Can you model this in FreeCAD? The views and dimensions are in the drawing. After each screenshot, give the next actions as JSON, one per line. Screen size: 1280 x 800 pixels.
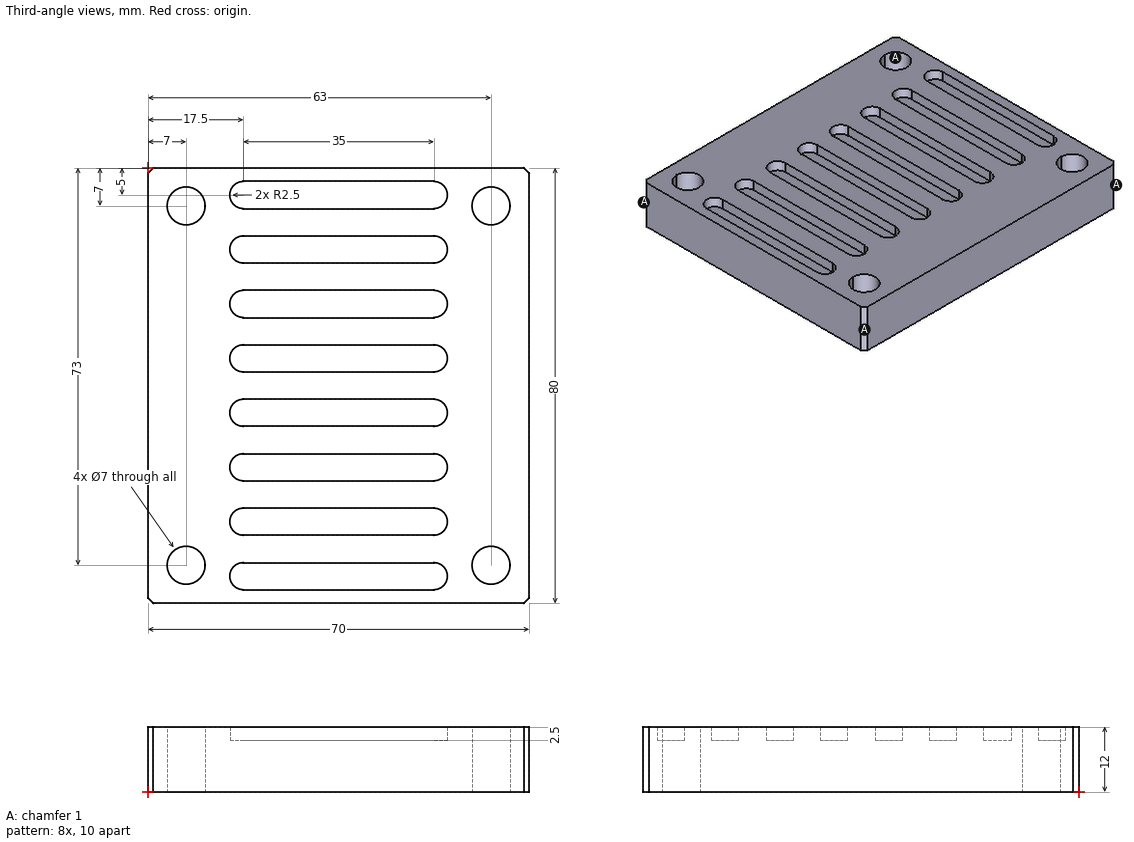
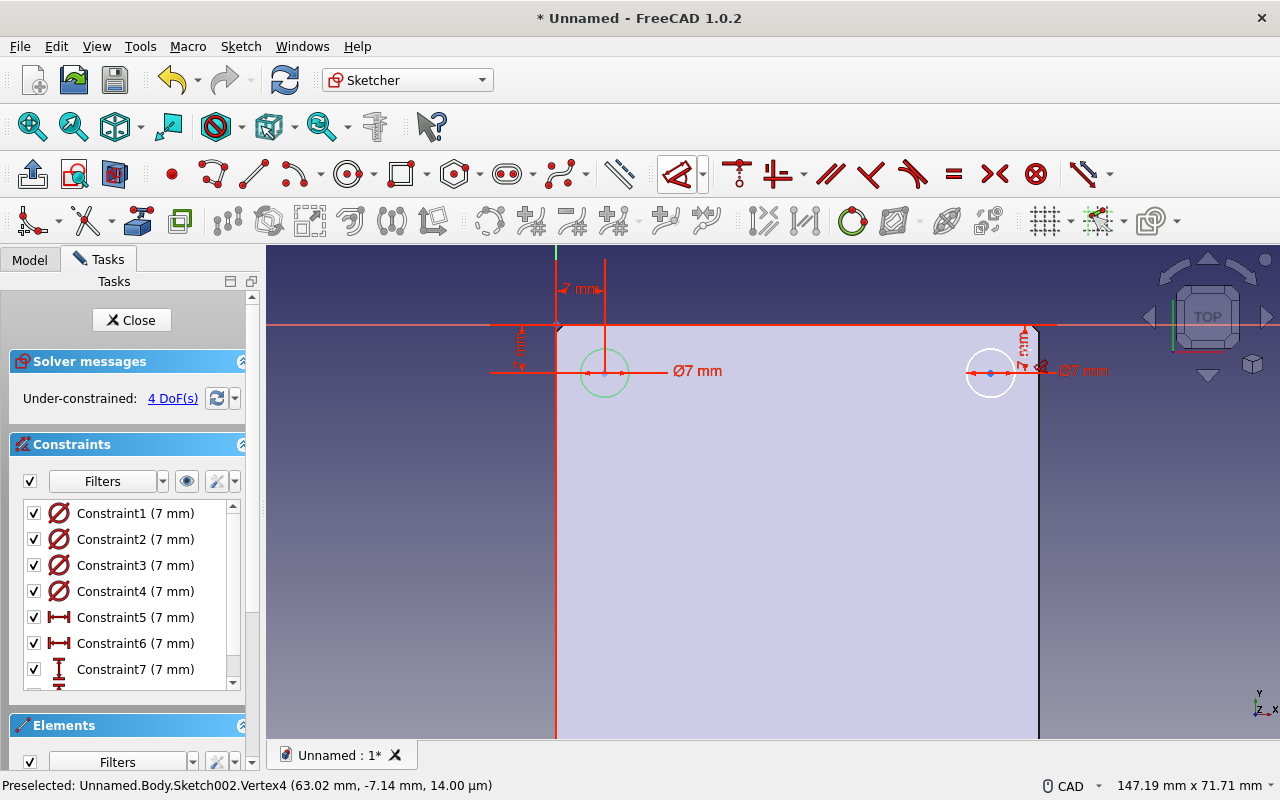
{"action": "scroll", "coordinate": [606, 375], "scroll_direction": "down", "scroll_amount": 3}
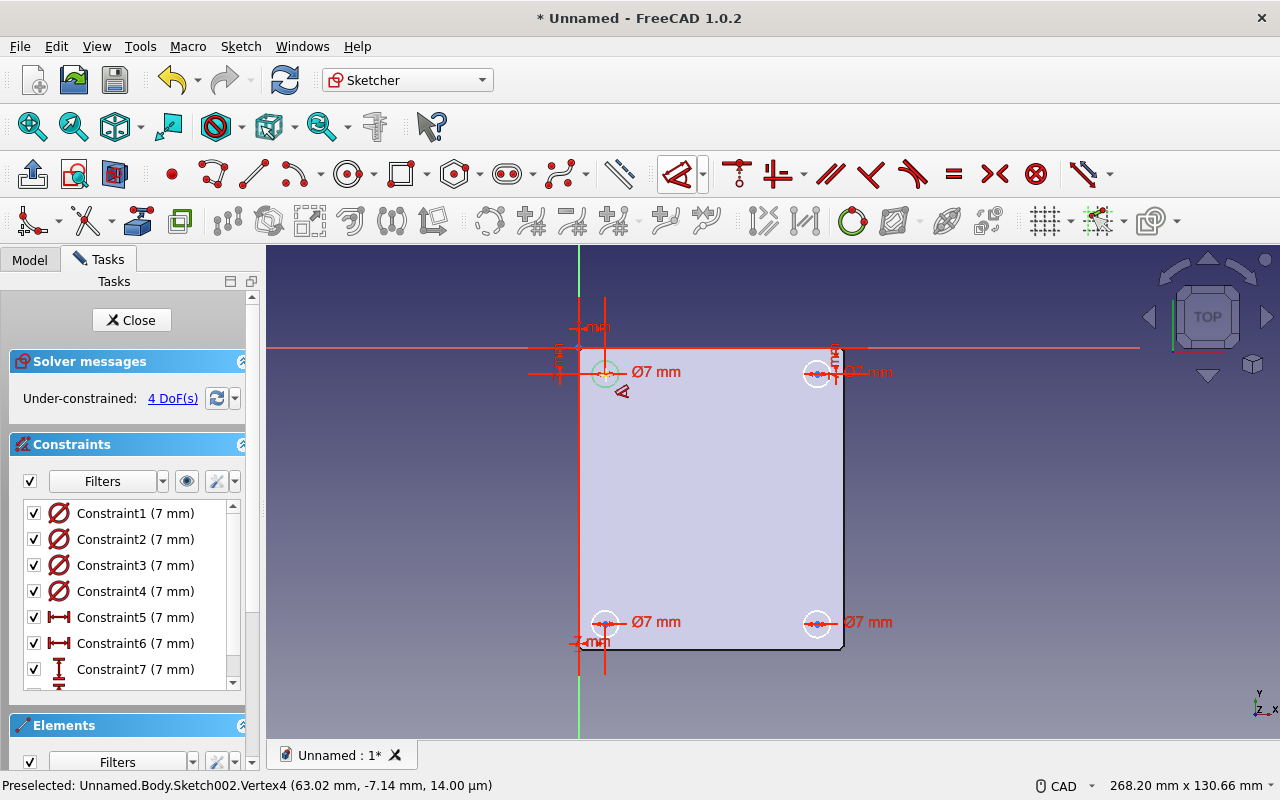
{"action": "left_click", "coordinate": [605, 624]}
{"action": "left_click", "coordinate": [545, 486]}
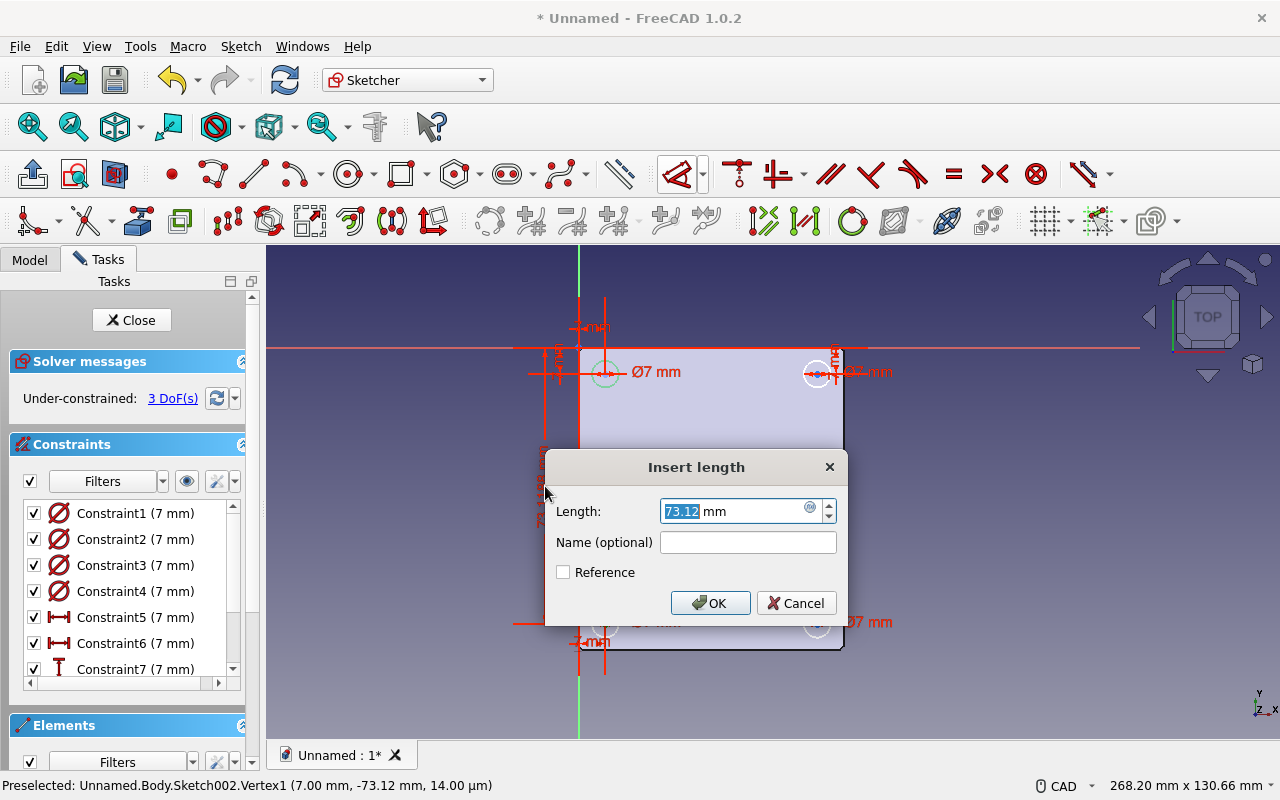
{"action": "type", "text": "73"}
{"action": "key", "text": "Return"}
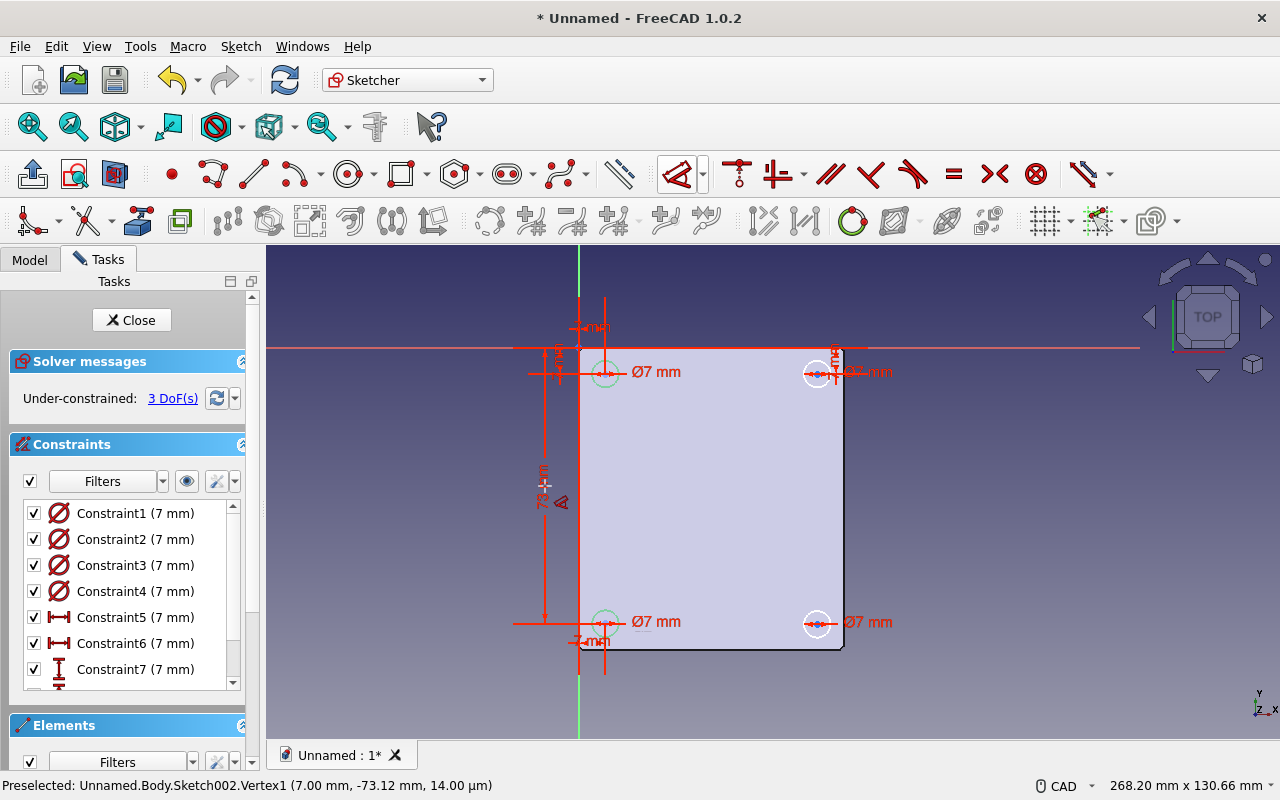
{"action": "left_click", "coordinate": [817, 624]}
{"action": "left_click", "coordinate": [698, 314]}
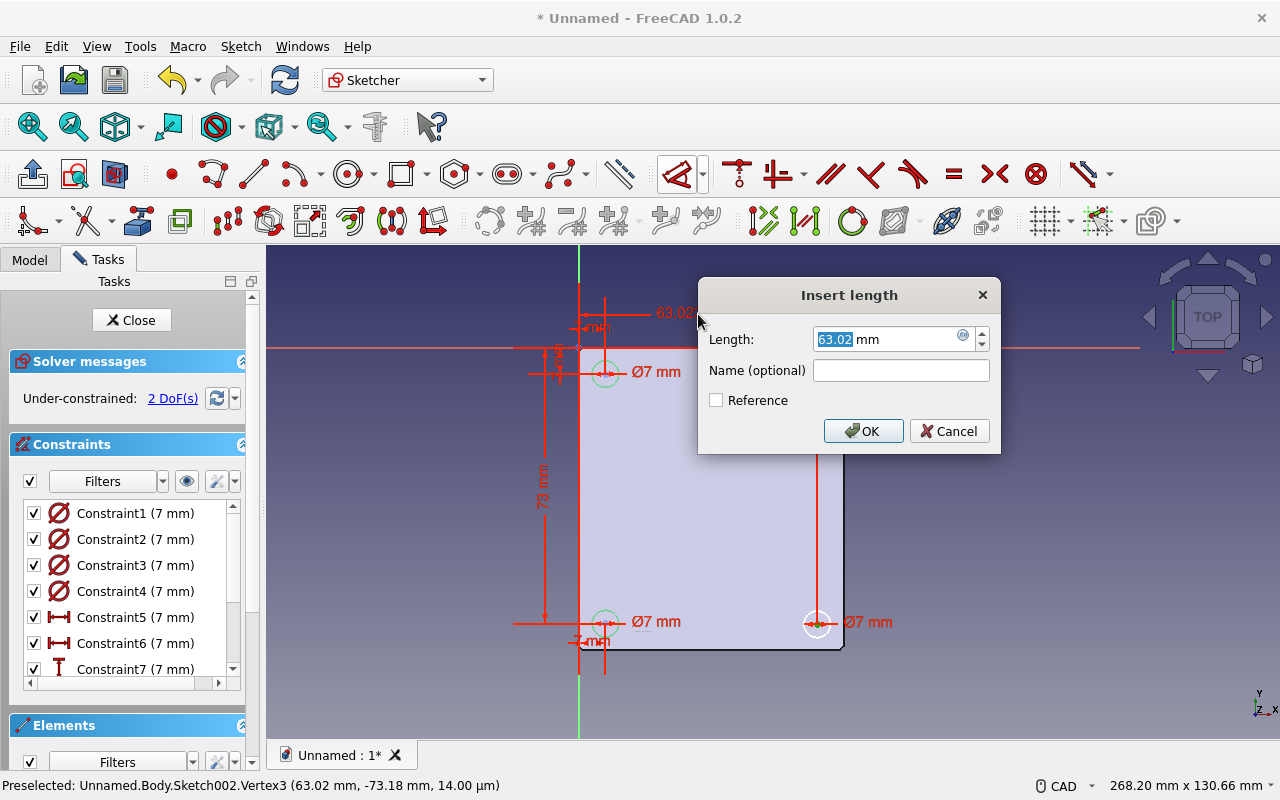
{"action": "type", "text": "63"}
{"action": "key", "text": "Return"}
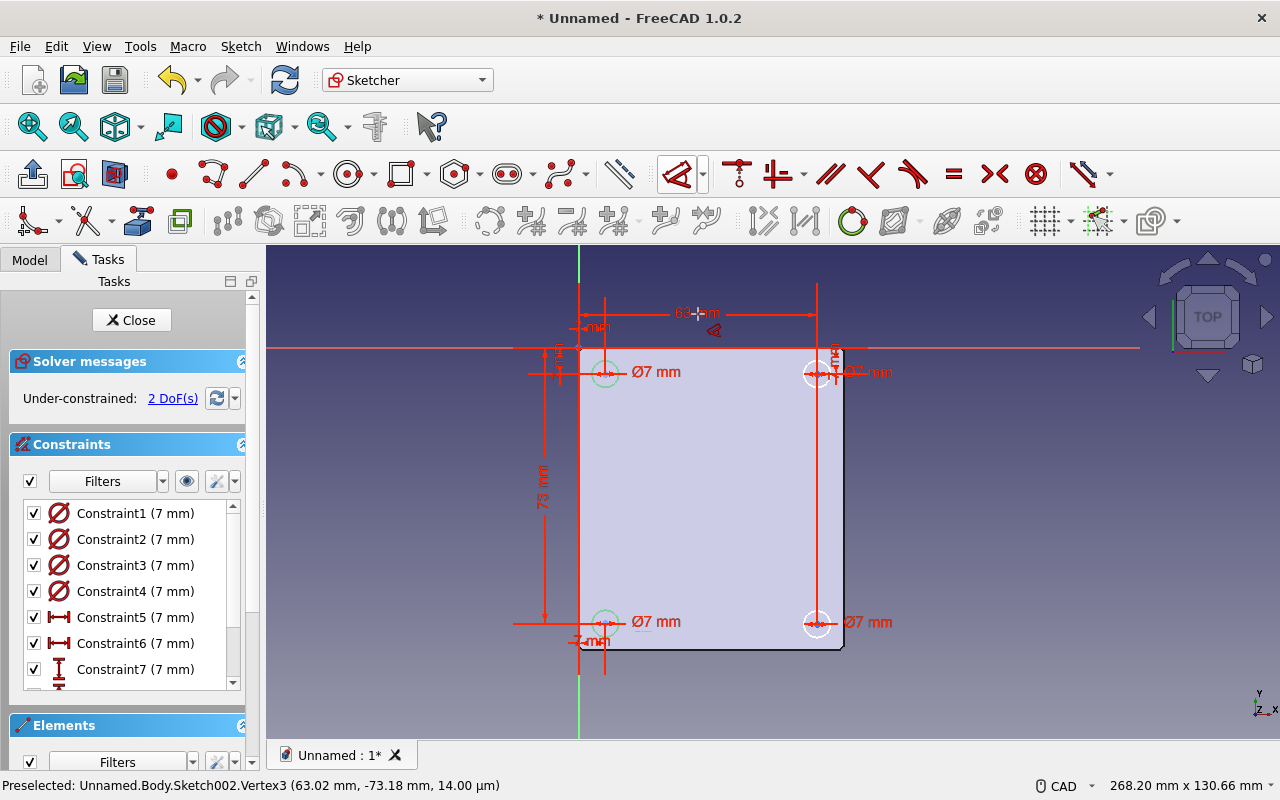
{"action": "left_click", "coordinate": [817, 624]}
{"action": "left_click", "coordinate": [545, 422]}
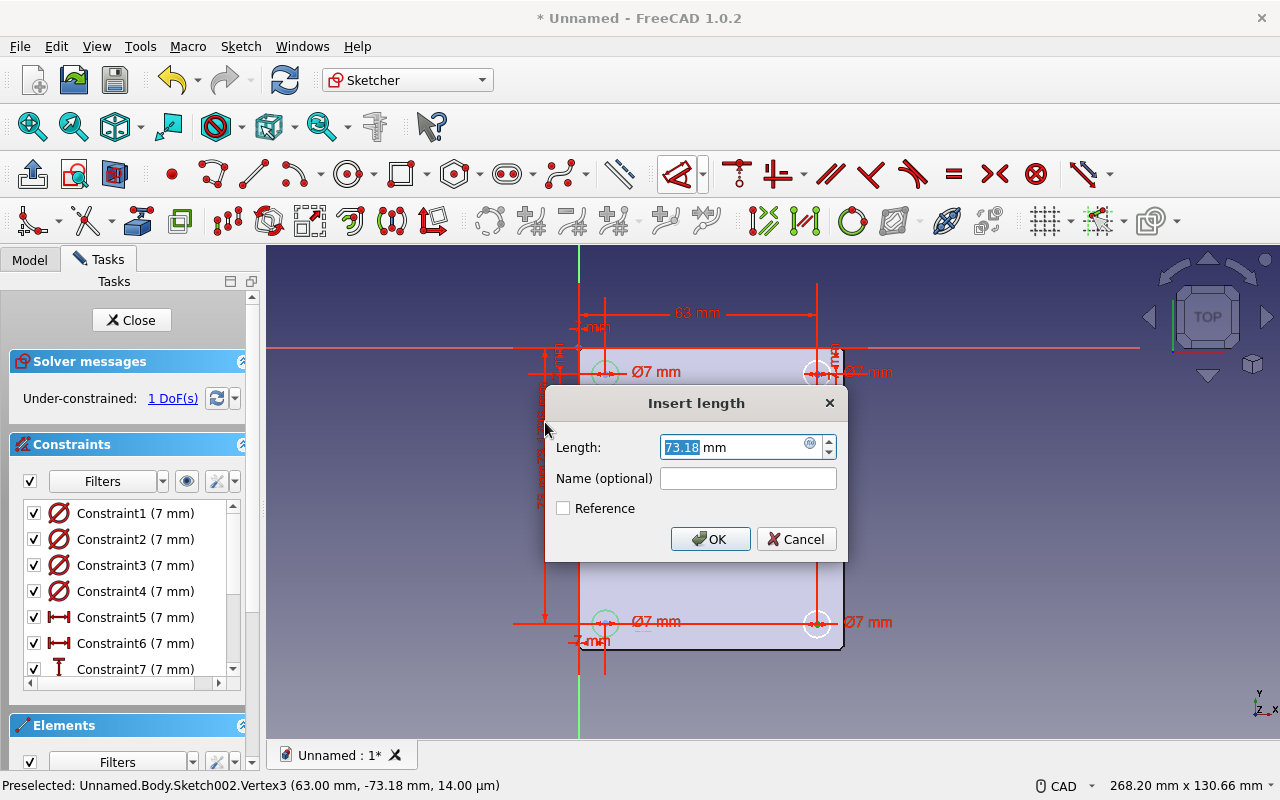
{"action": "type", "text": "73"}
{"action": "key", "text": "Return"}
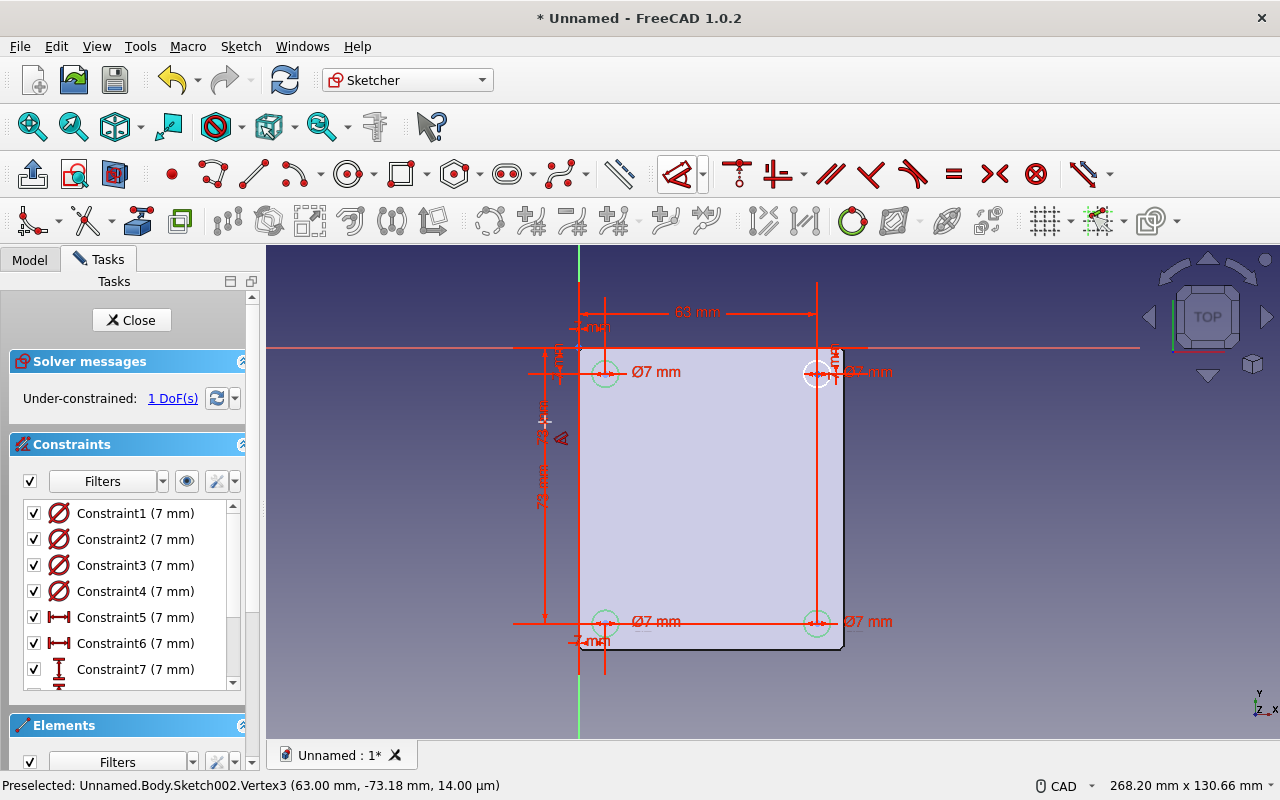
{"action": "left_click", "coordinate": [817, 374]}
{"action": "left_click", "coordinate": [782, 314]}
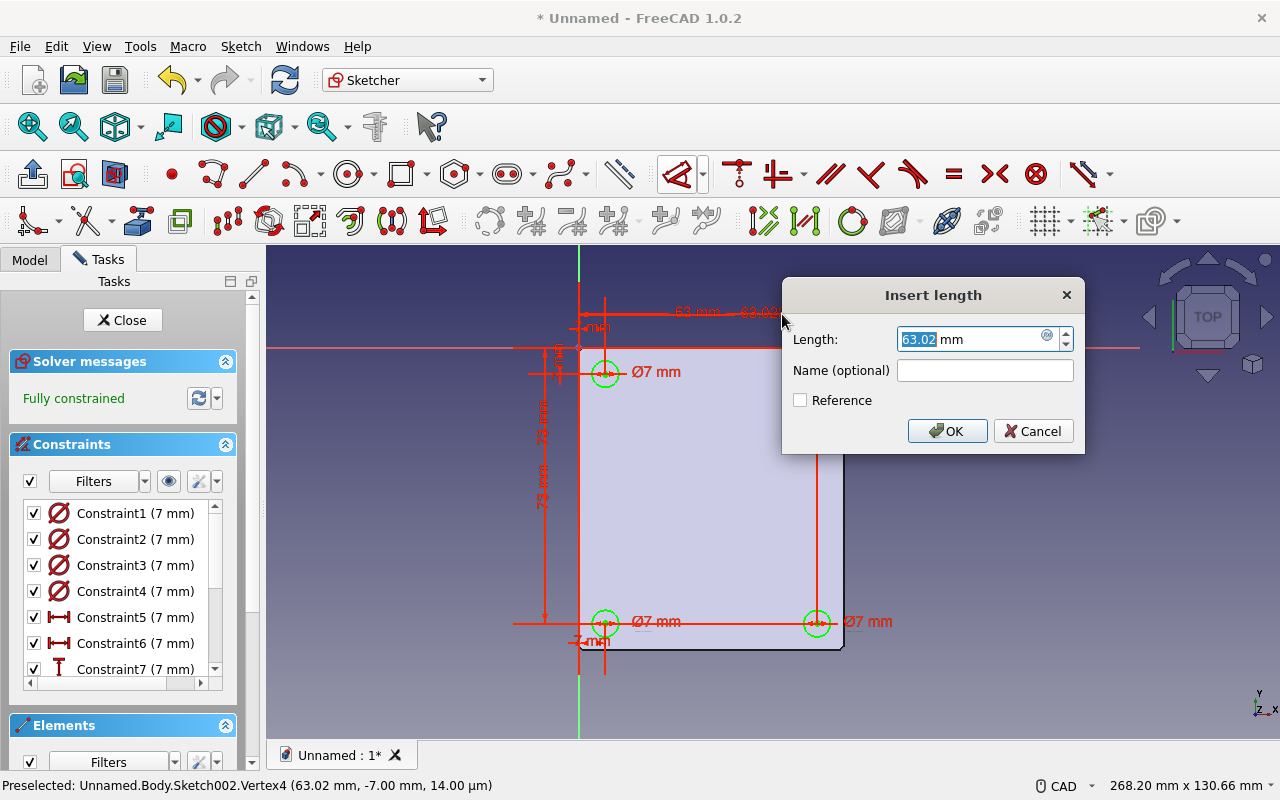
{"action": "type", "text": "63"}
{"action": "key", "text": "Return"}
{"action": "key", "text": "Escape"}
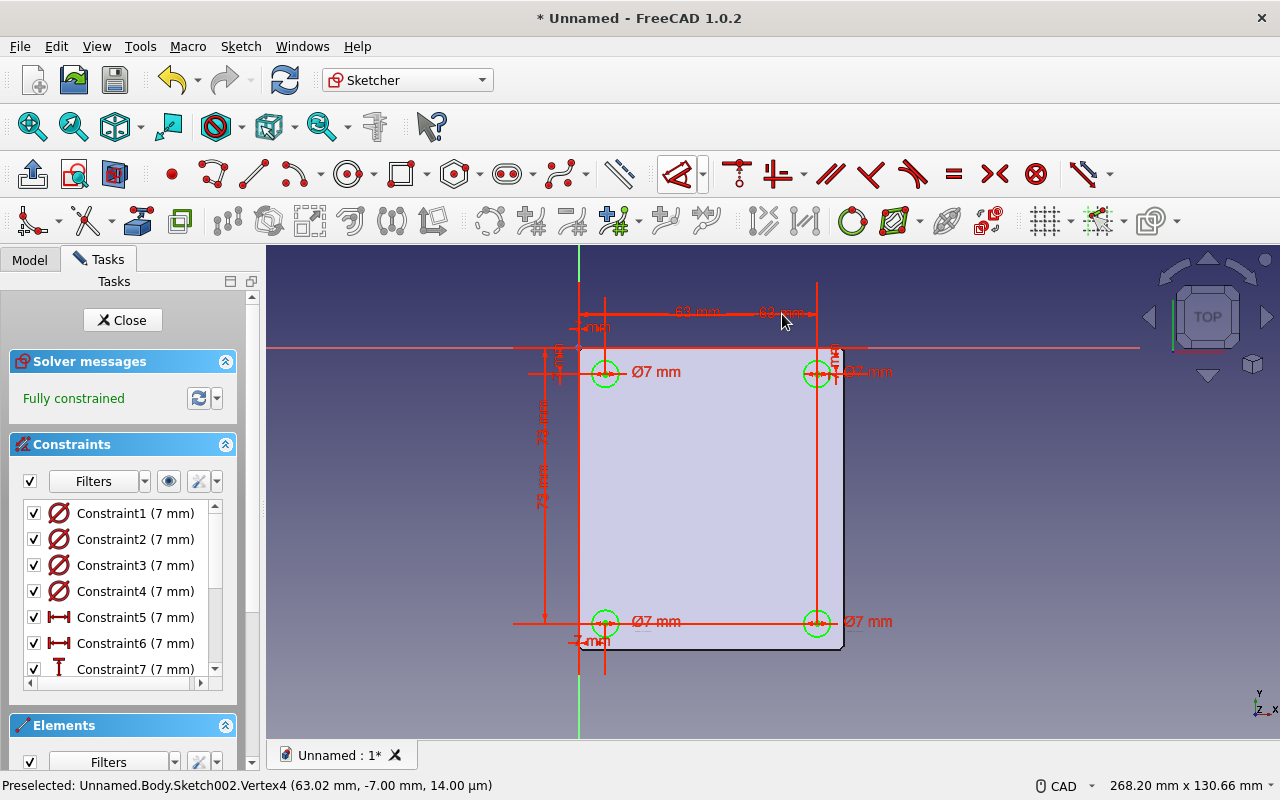
{"action": "left_click", "coordinate": [123, 320]}